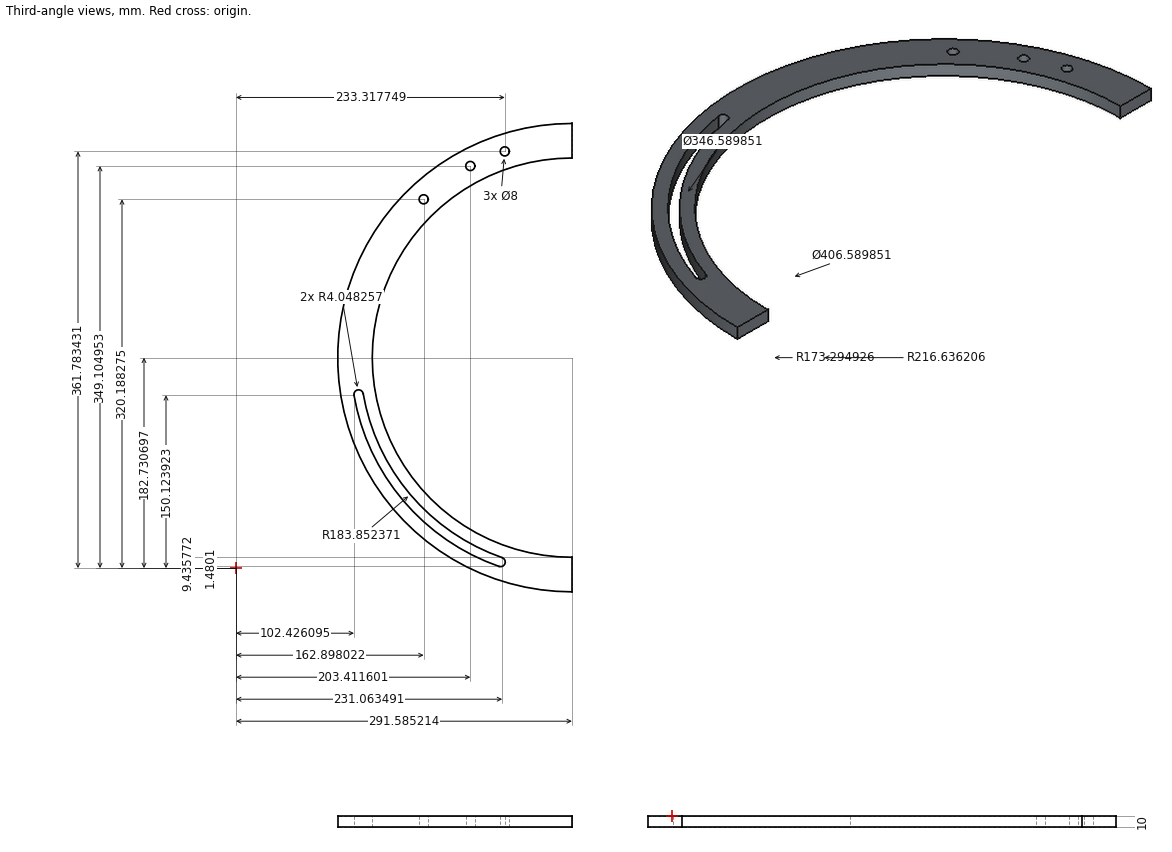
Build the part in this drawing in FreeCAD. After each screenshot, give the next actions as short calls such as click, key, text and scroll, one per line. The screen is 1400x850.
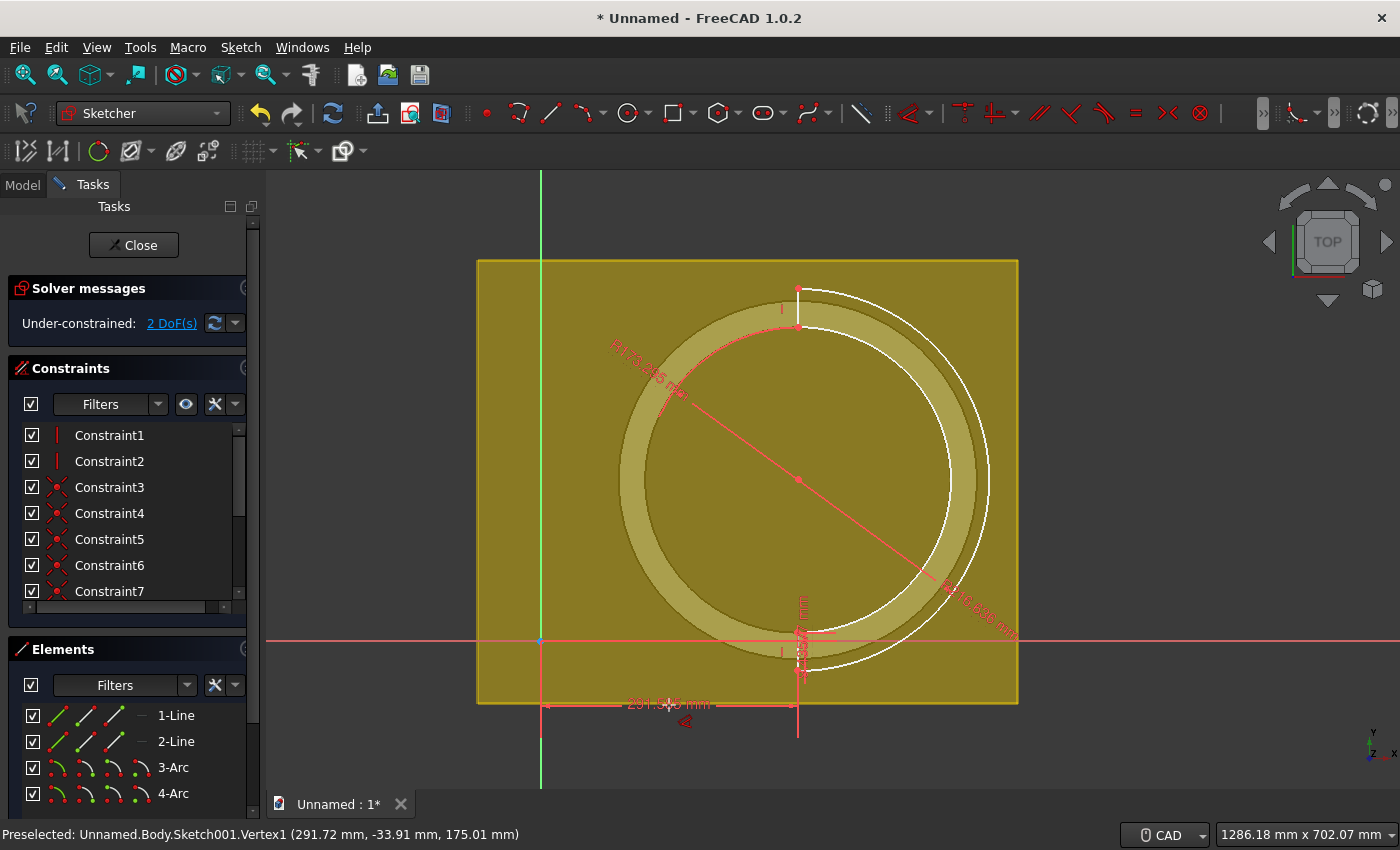
click(798, 327)
click(669, 675)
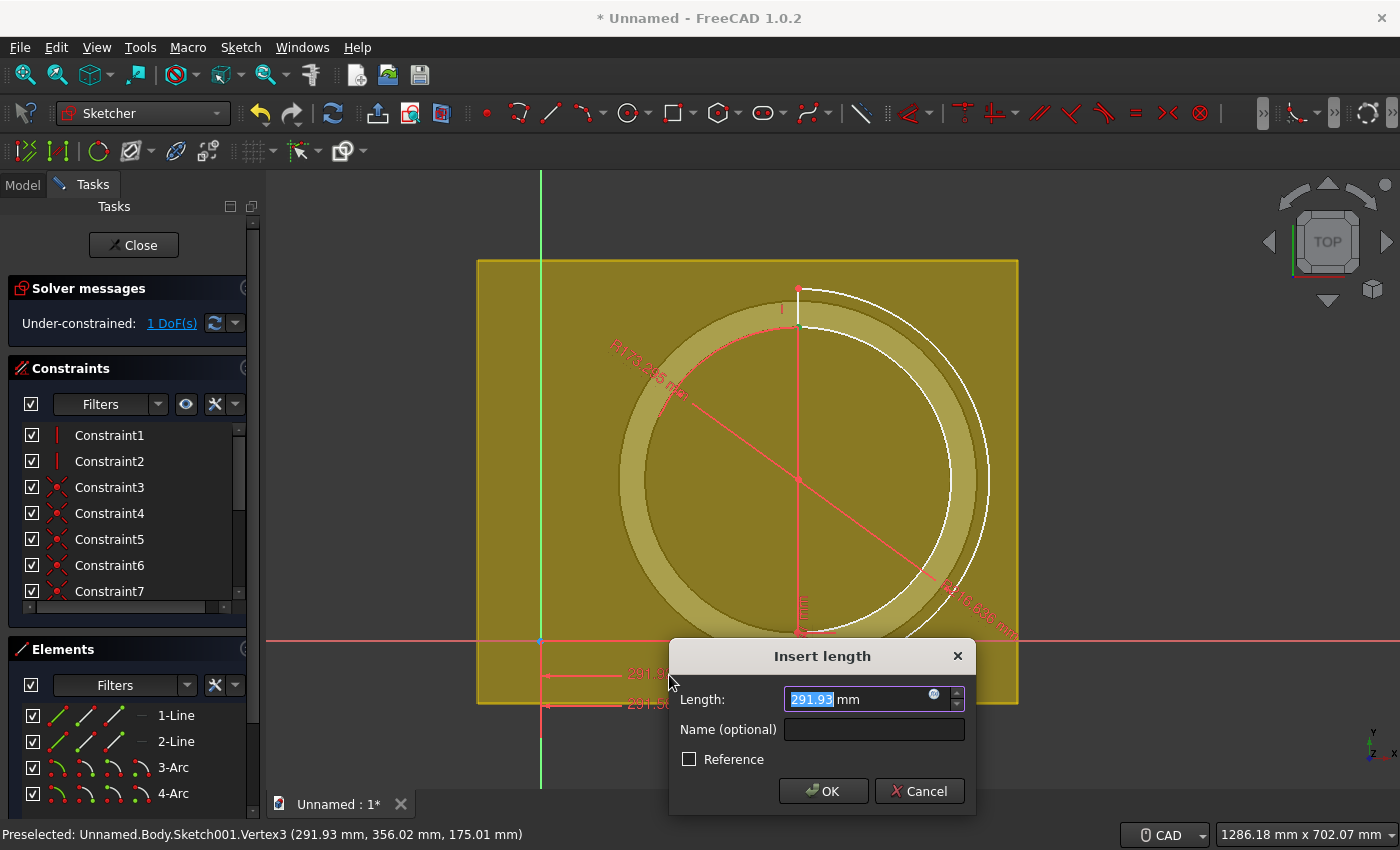
text(291.585214)
key(Return)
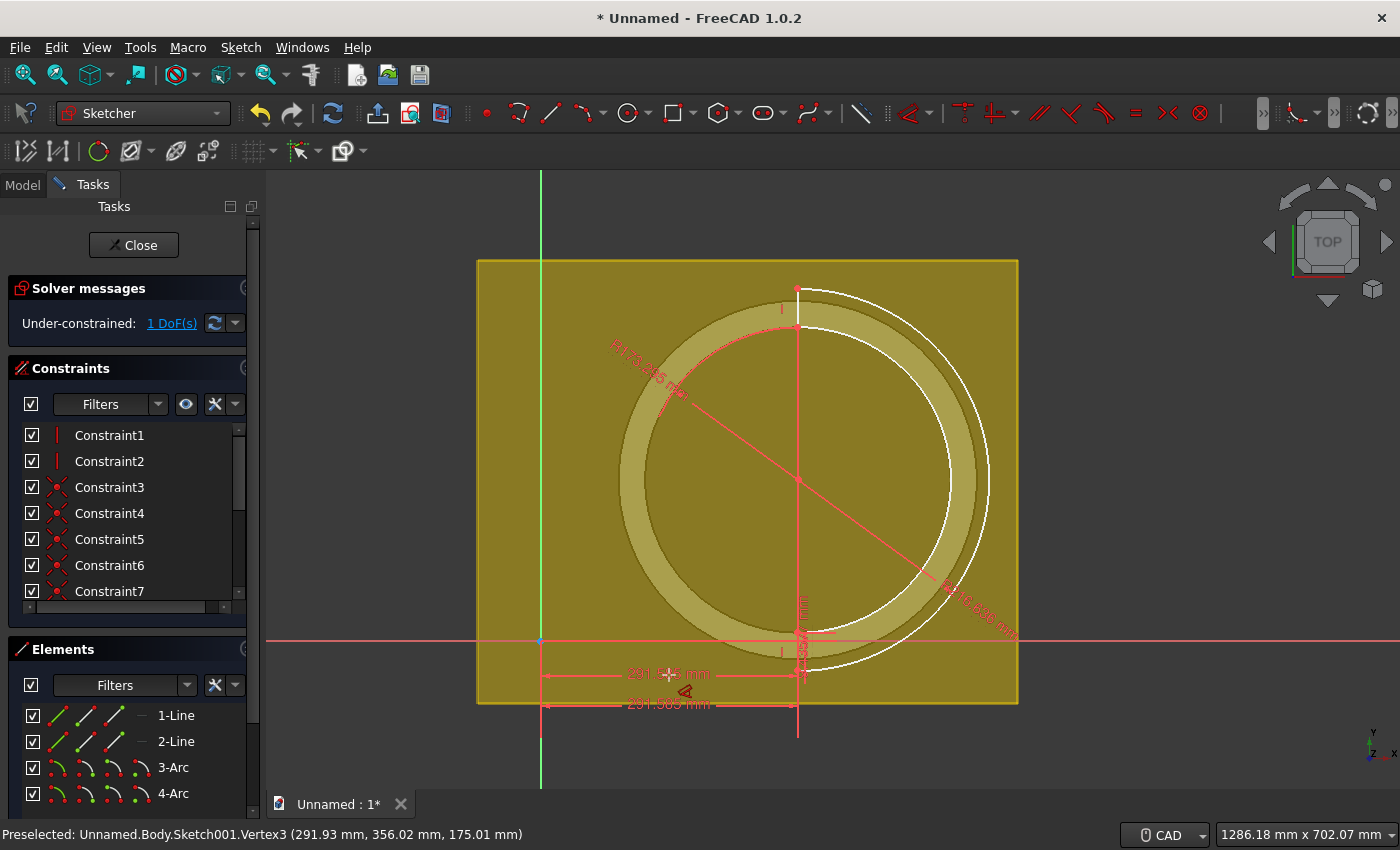
click(798, 480)
click(579, 675)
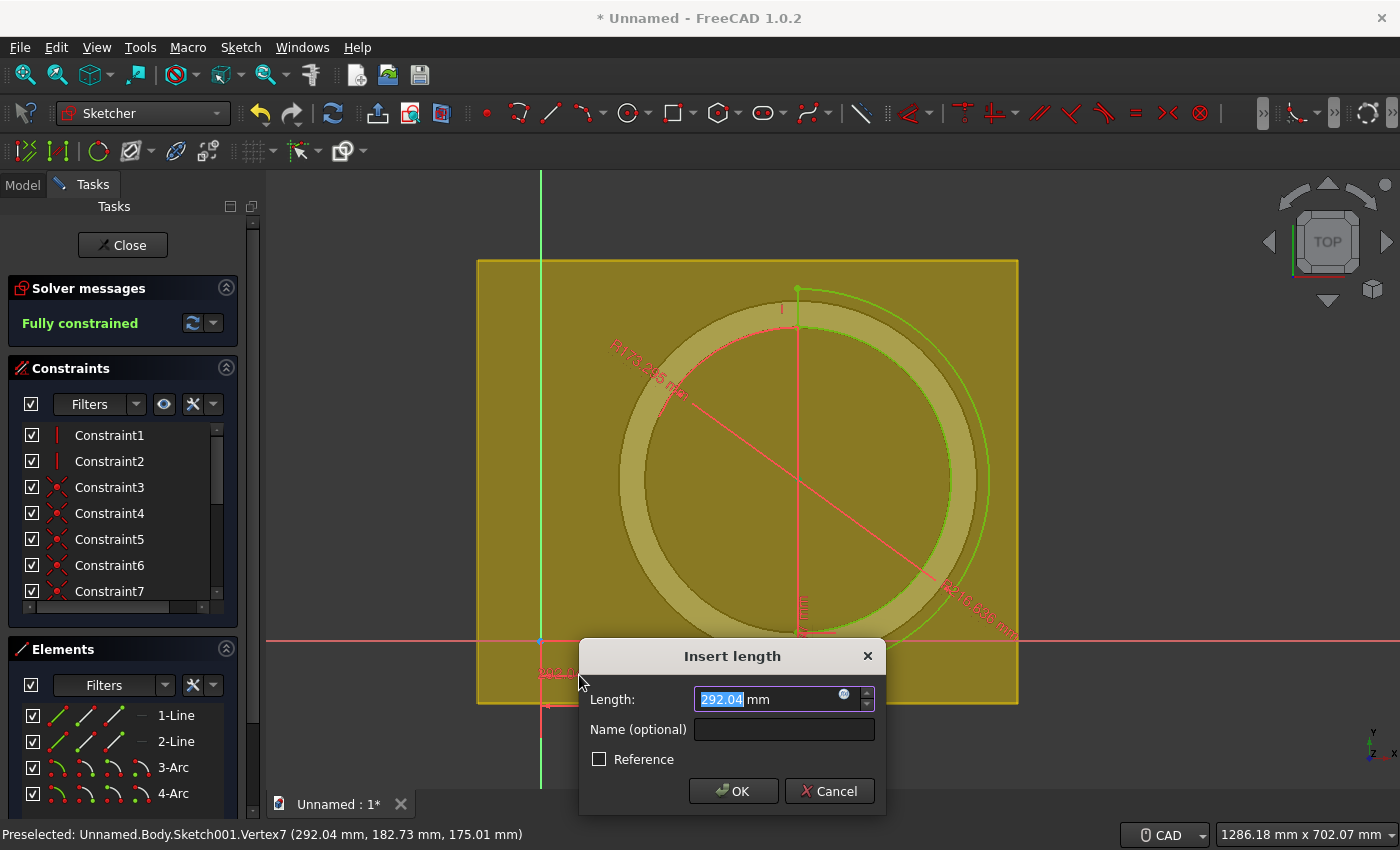
text(291.585214)
key(Return)
key(Escape)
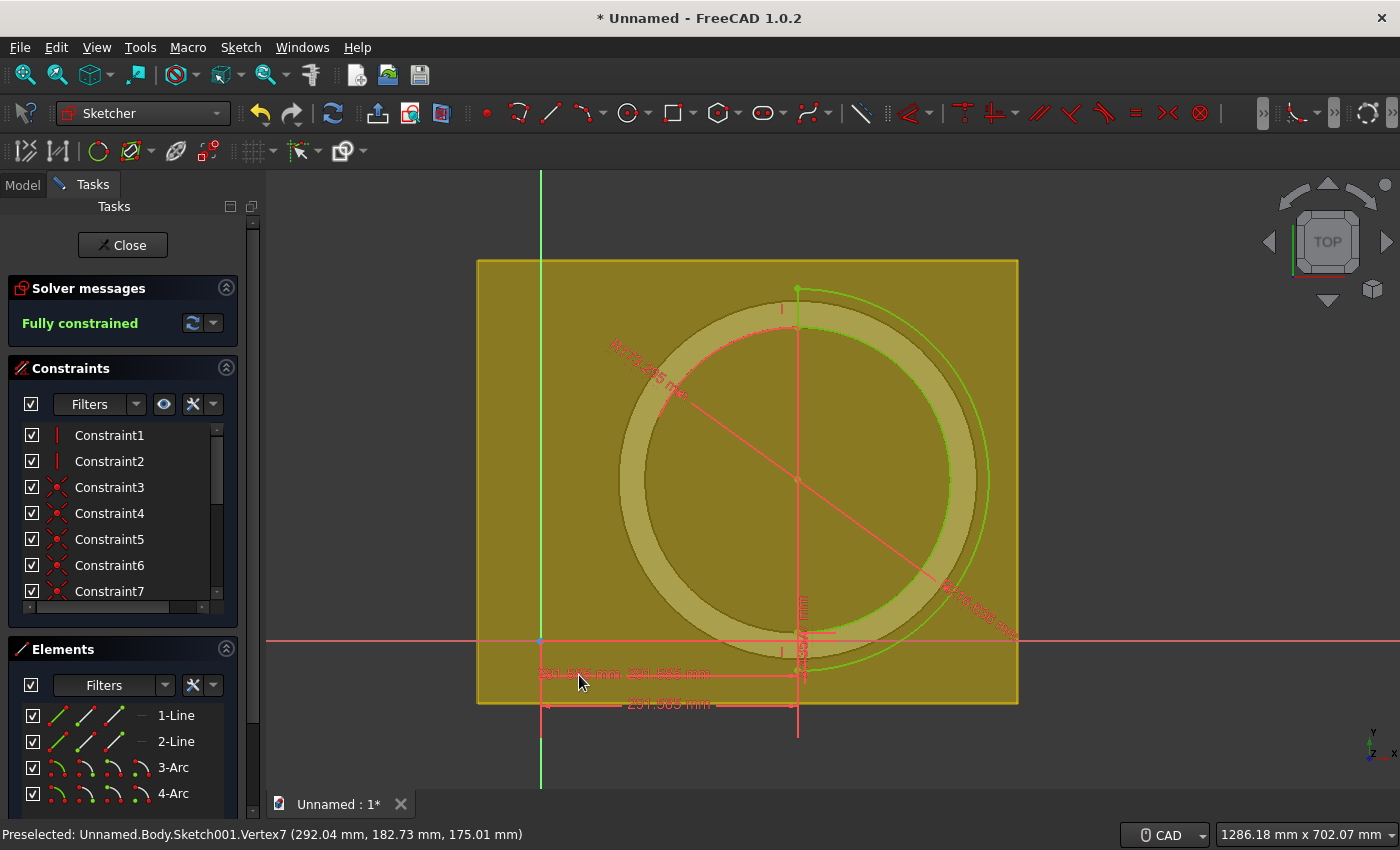
click(123, 245)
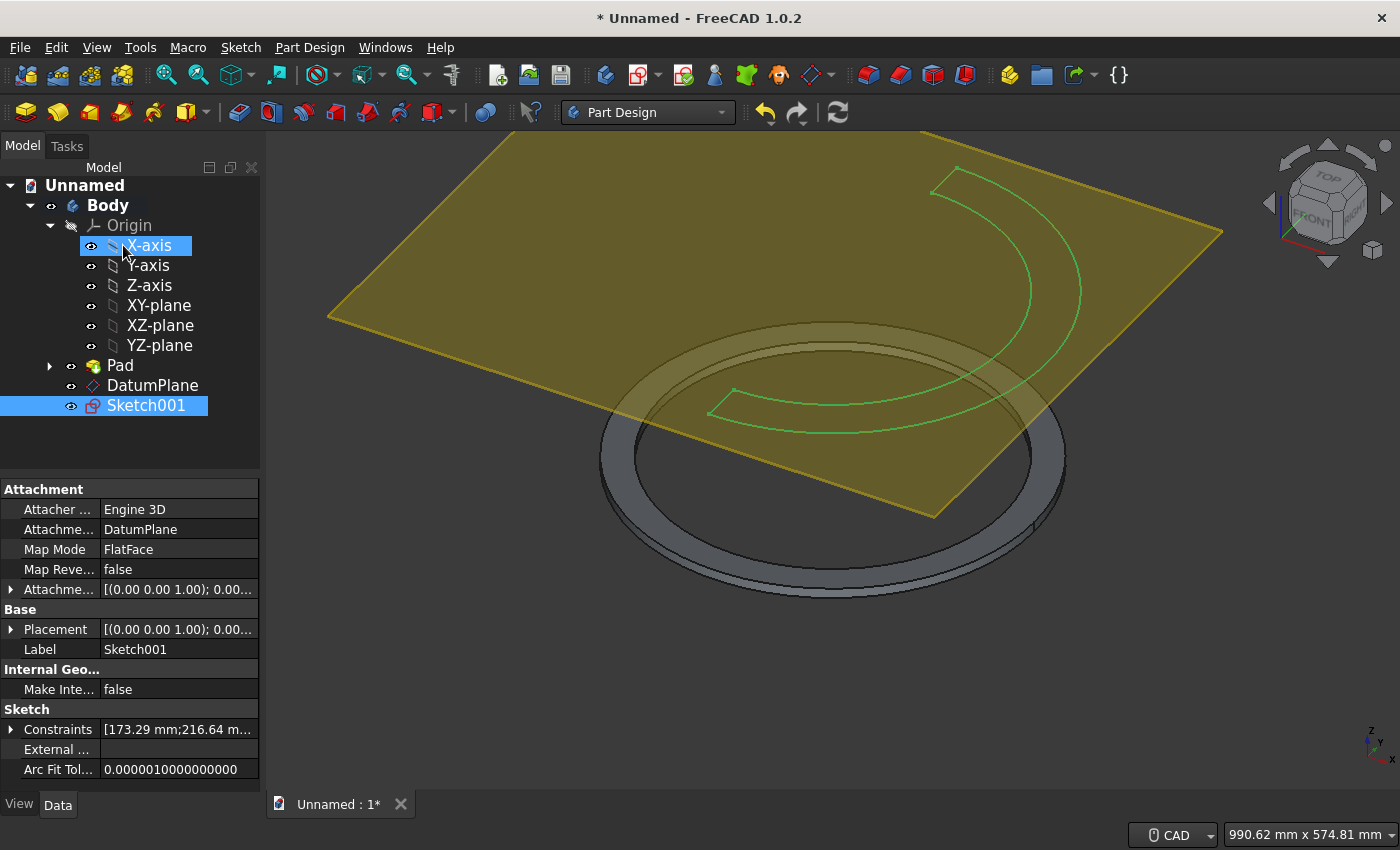
click(240, 112)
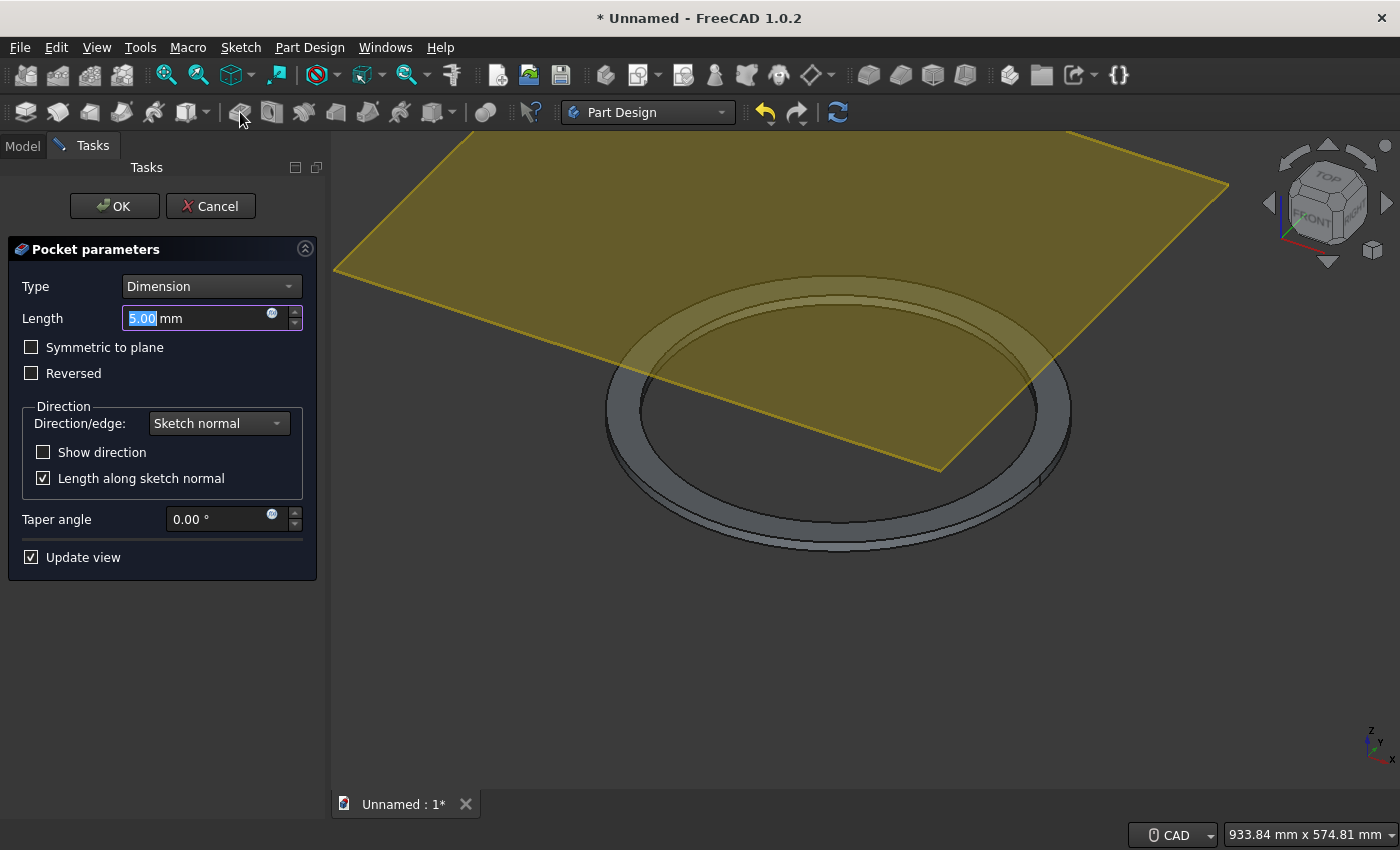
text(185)
key(Tab)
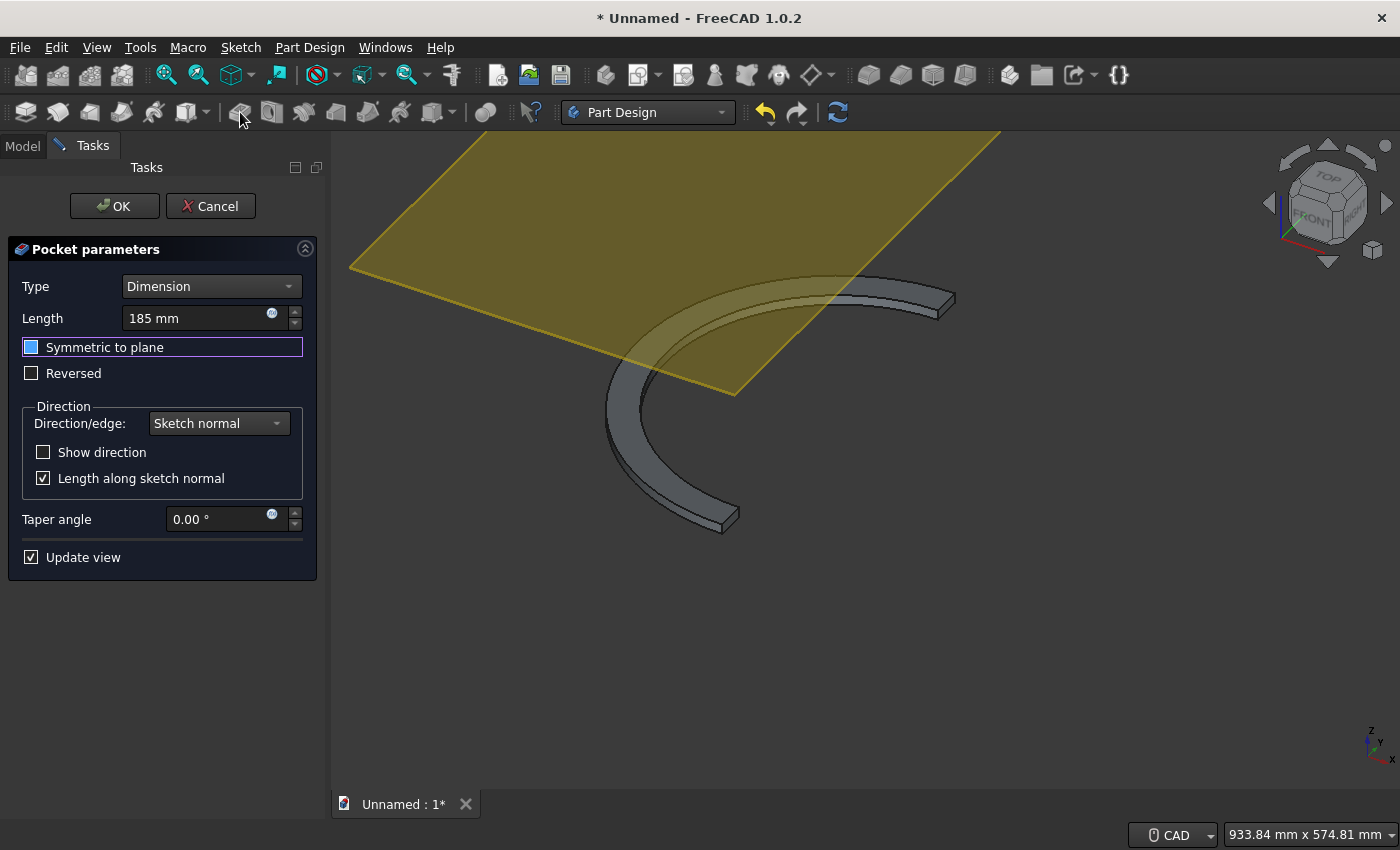
click(115, 206)